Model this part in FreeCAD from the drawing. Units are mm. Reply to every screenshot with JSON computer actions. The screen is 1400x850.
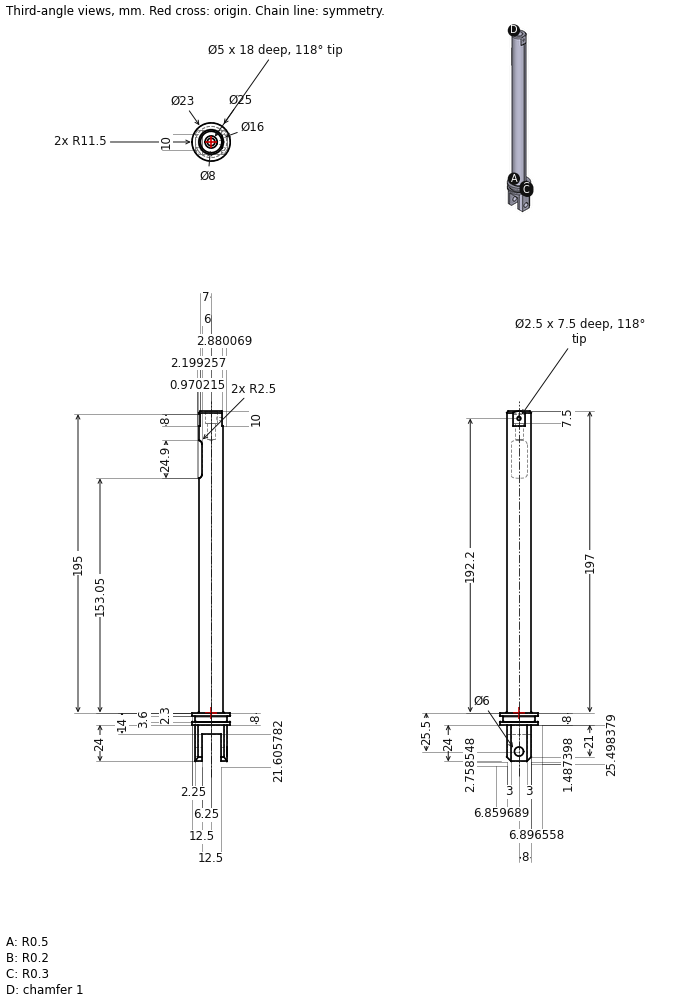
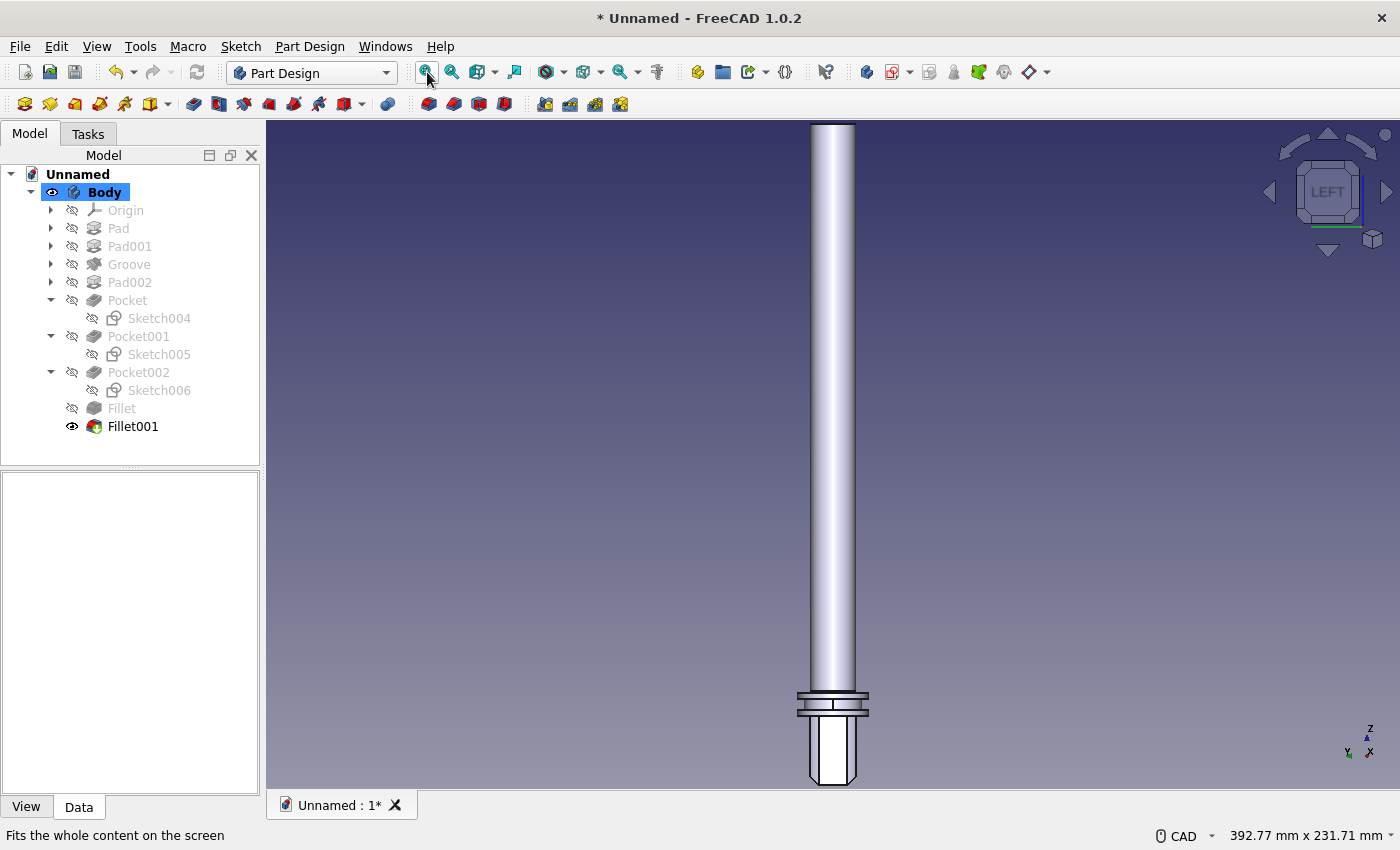
{"action": "key", "text": "v 3"}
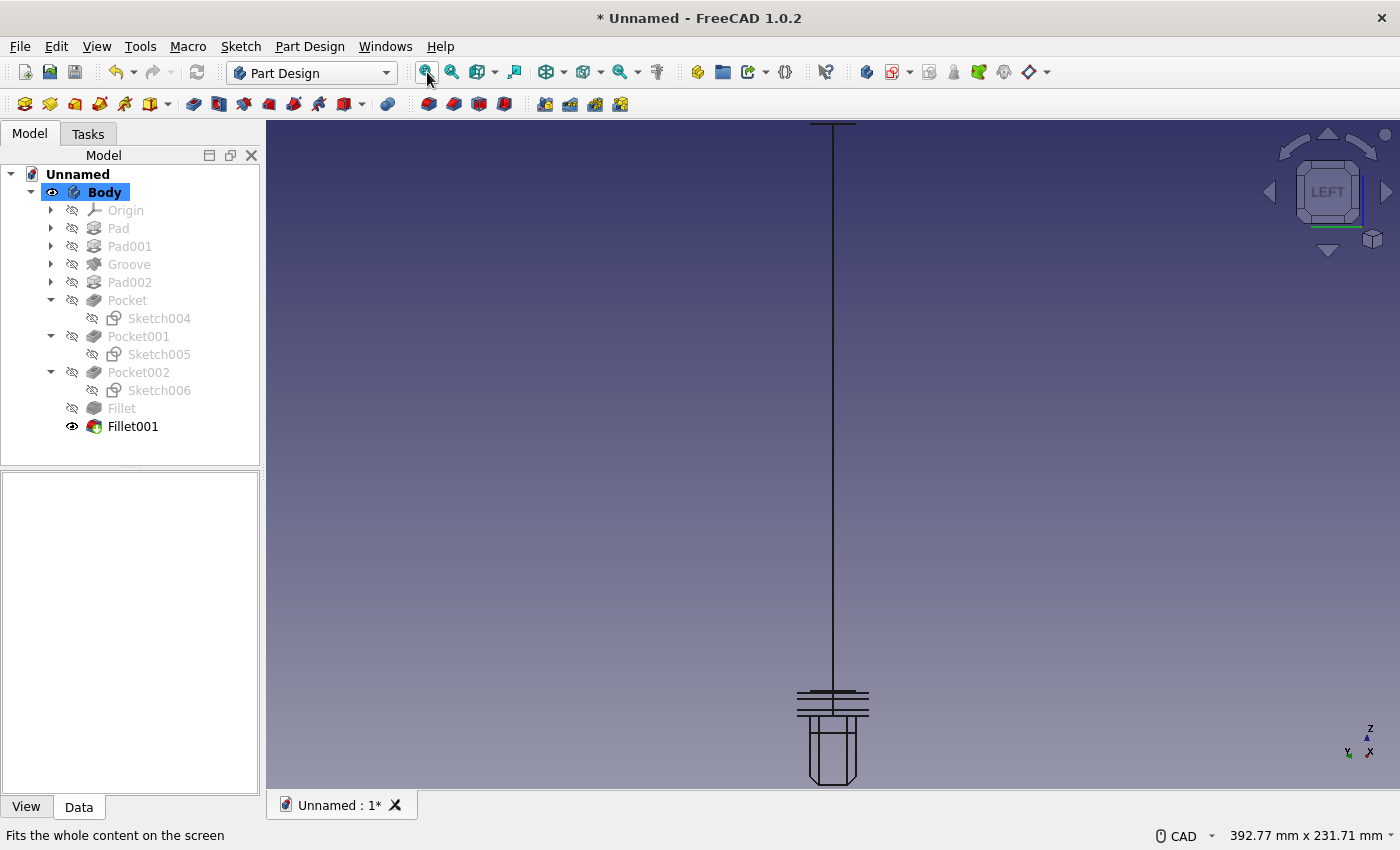
{"action": "key", "text": "0"}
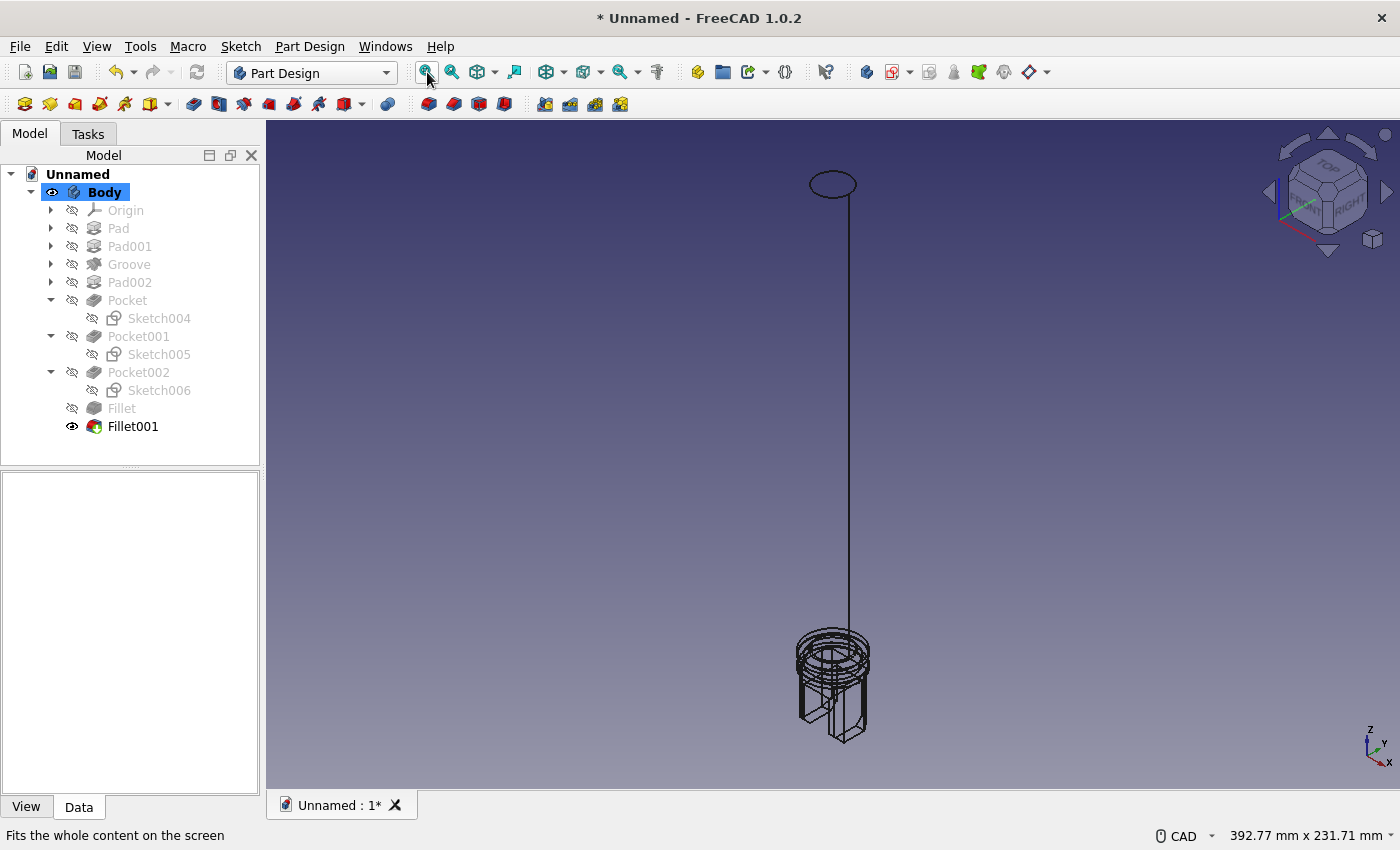
{"action": "left_click", "coordinate": [832, 645]}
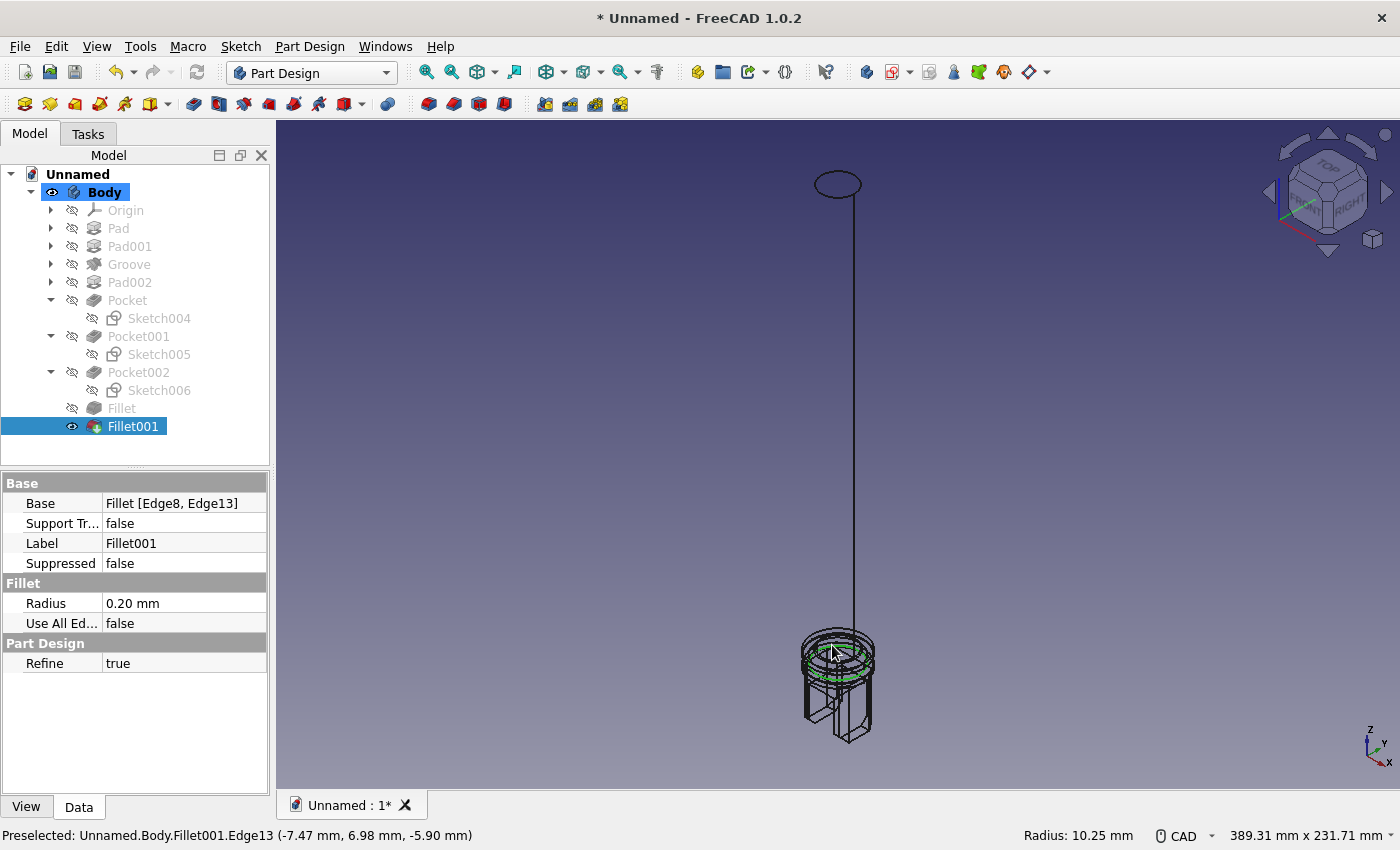
{"action": "scroll", "coordinate": [859, 665], "scroll_direction": "up", "scroll_amount": 6}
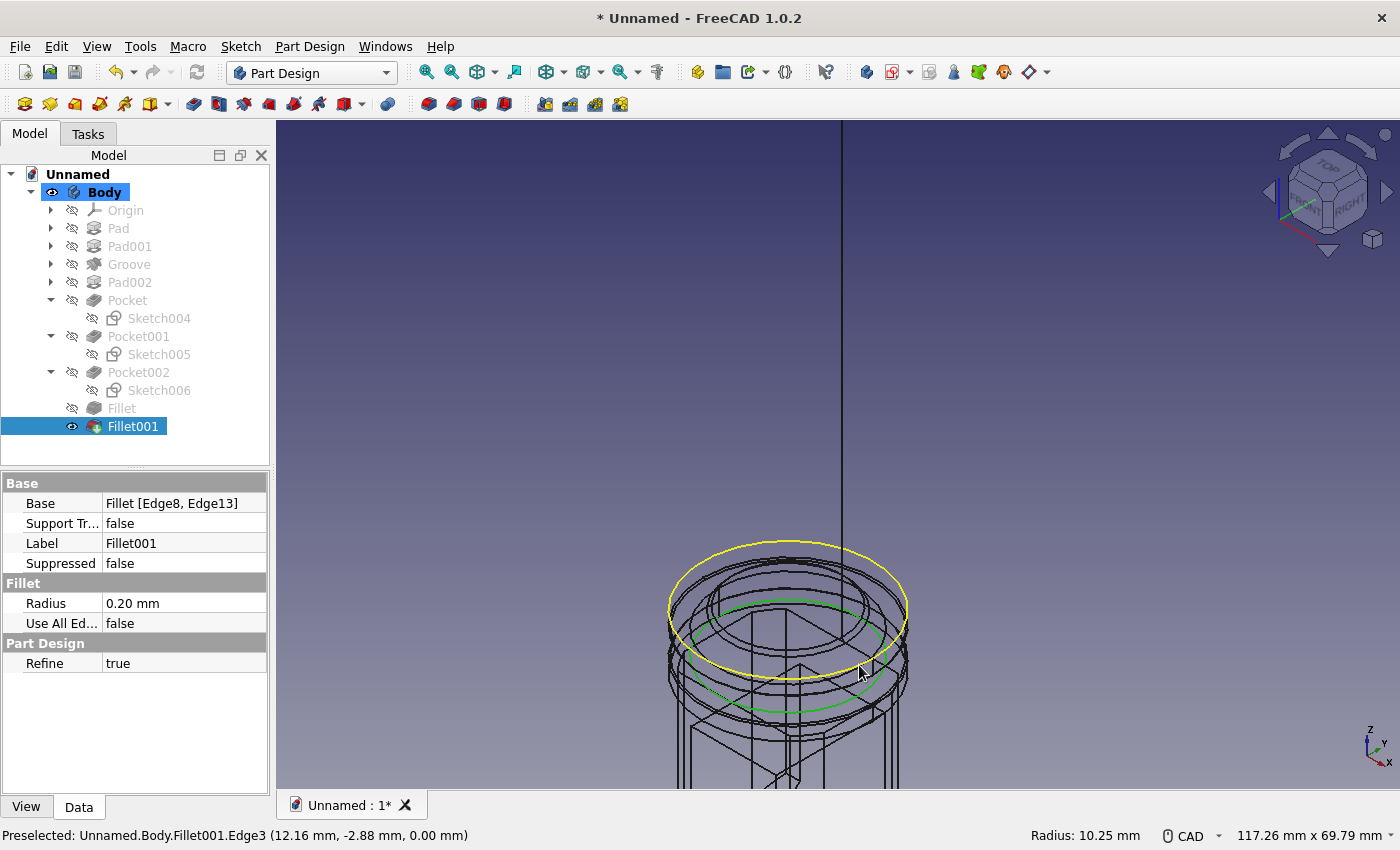
{"action": "left_click", "coordinate": [885, 636], "text": "ctrl"}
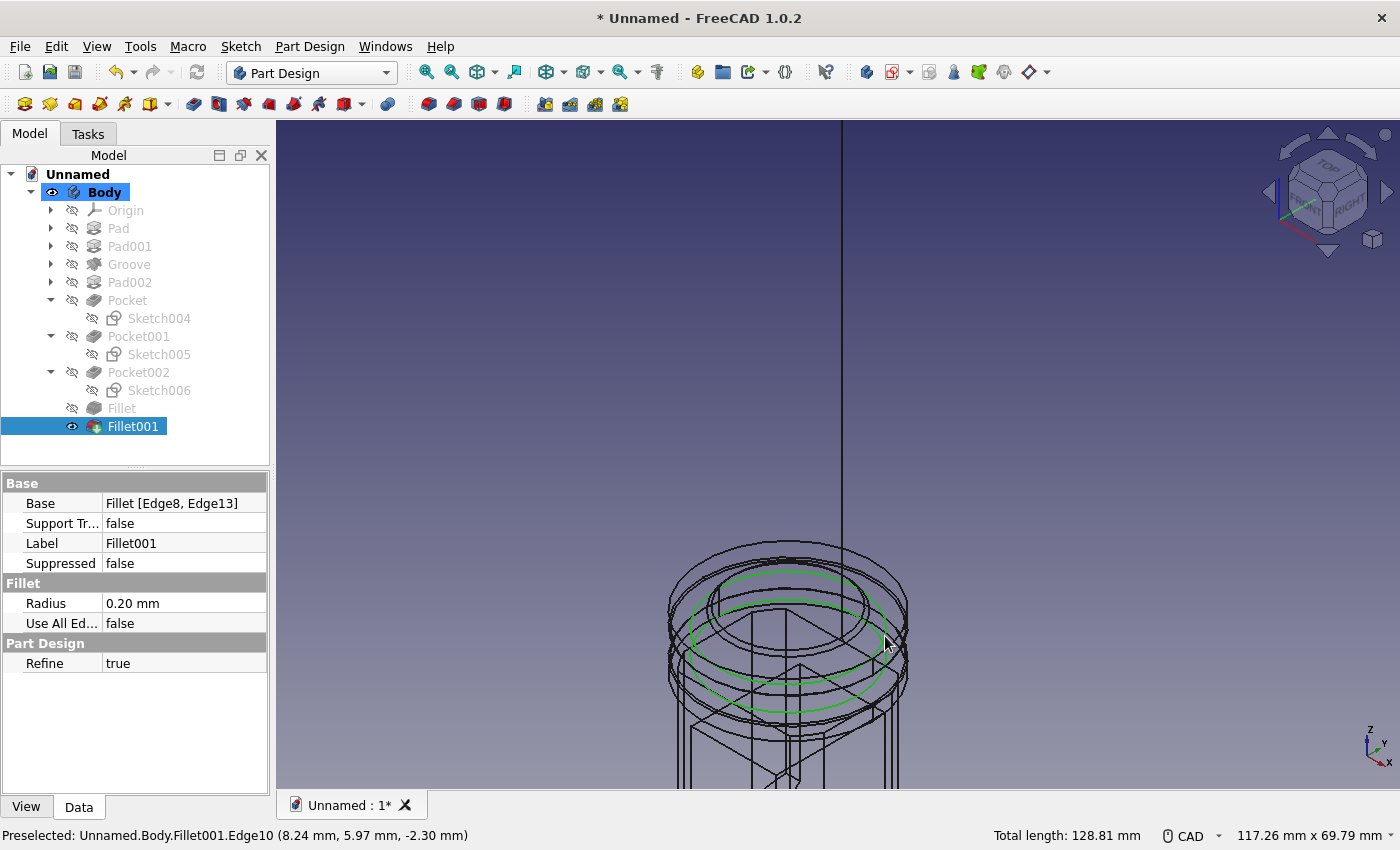
{"action": "key", "text": "v 1"}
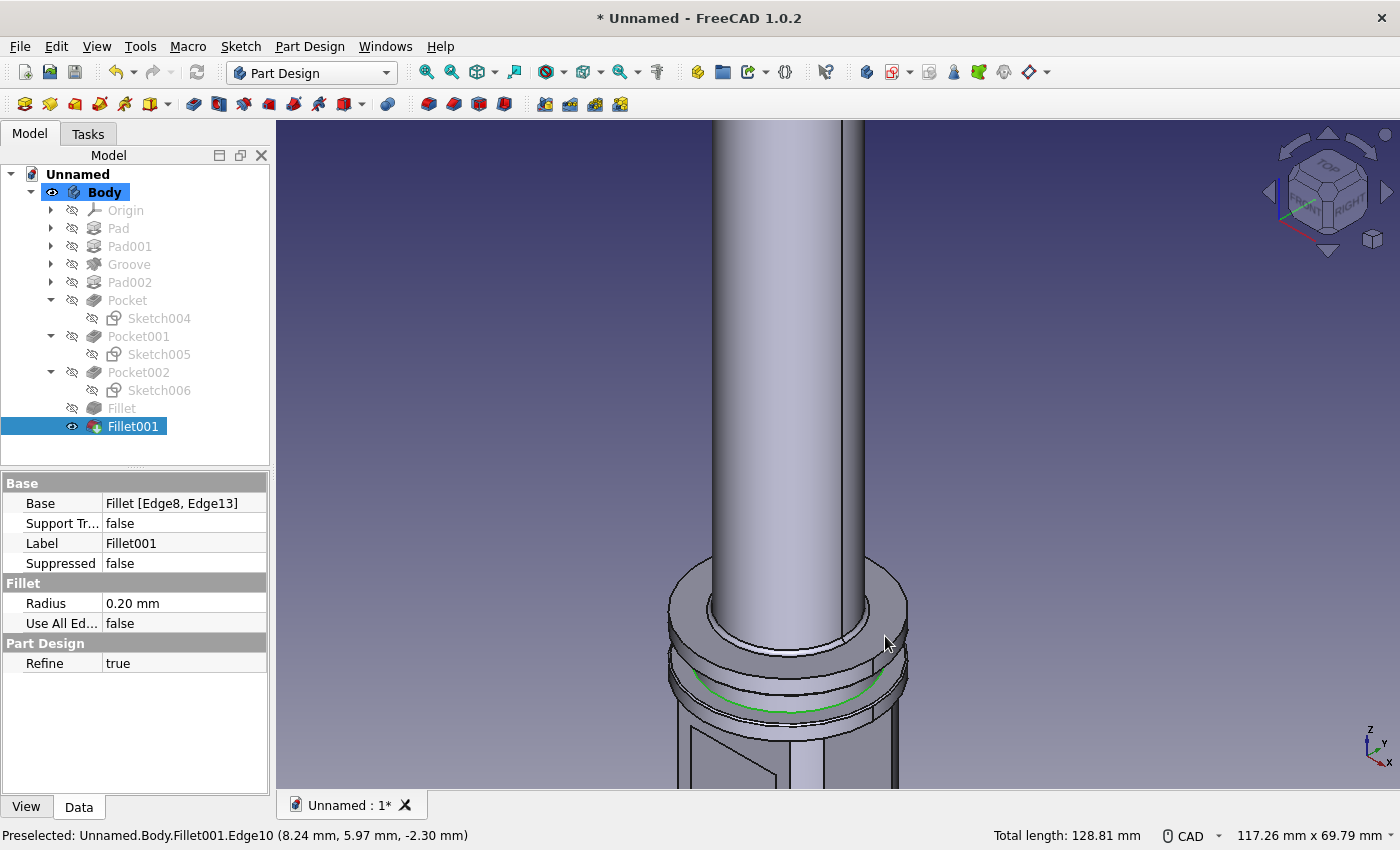
{"action": "left_click", "coordinate": [429, 104]}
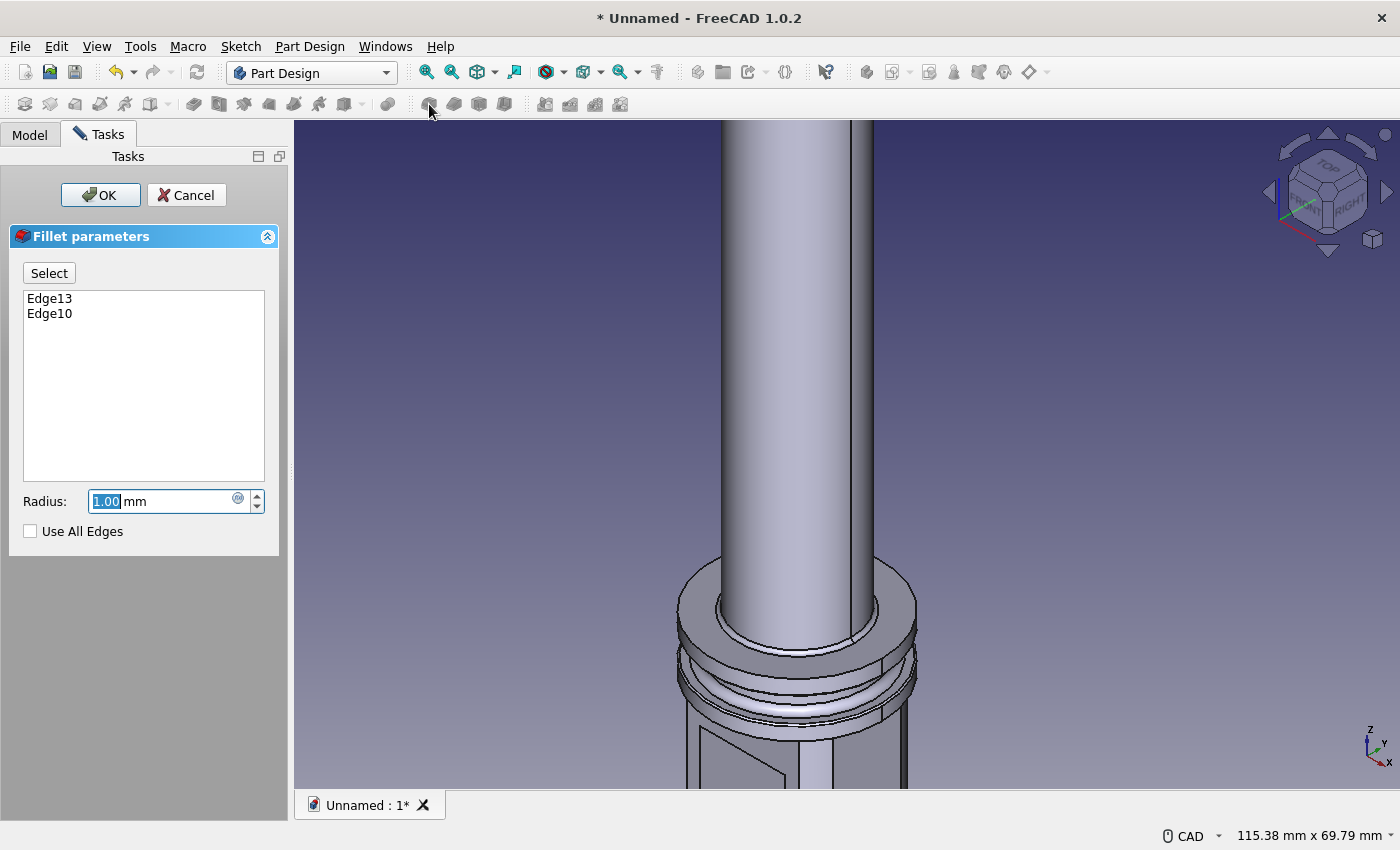
{"action": "type", "text": "0.3"}
{"action": "key", "text": "Tab"}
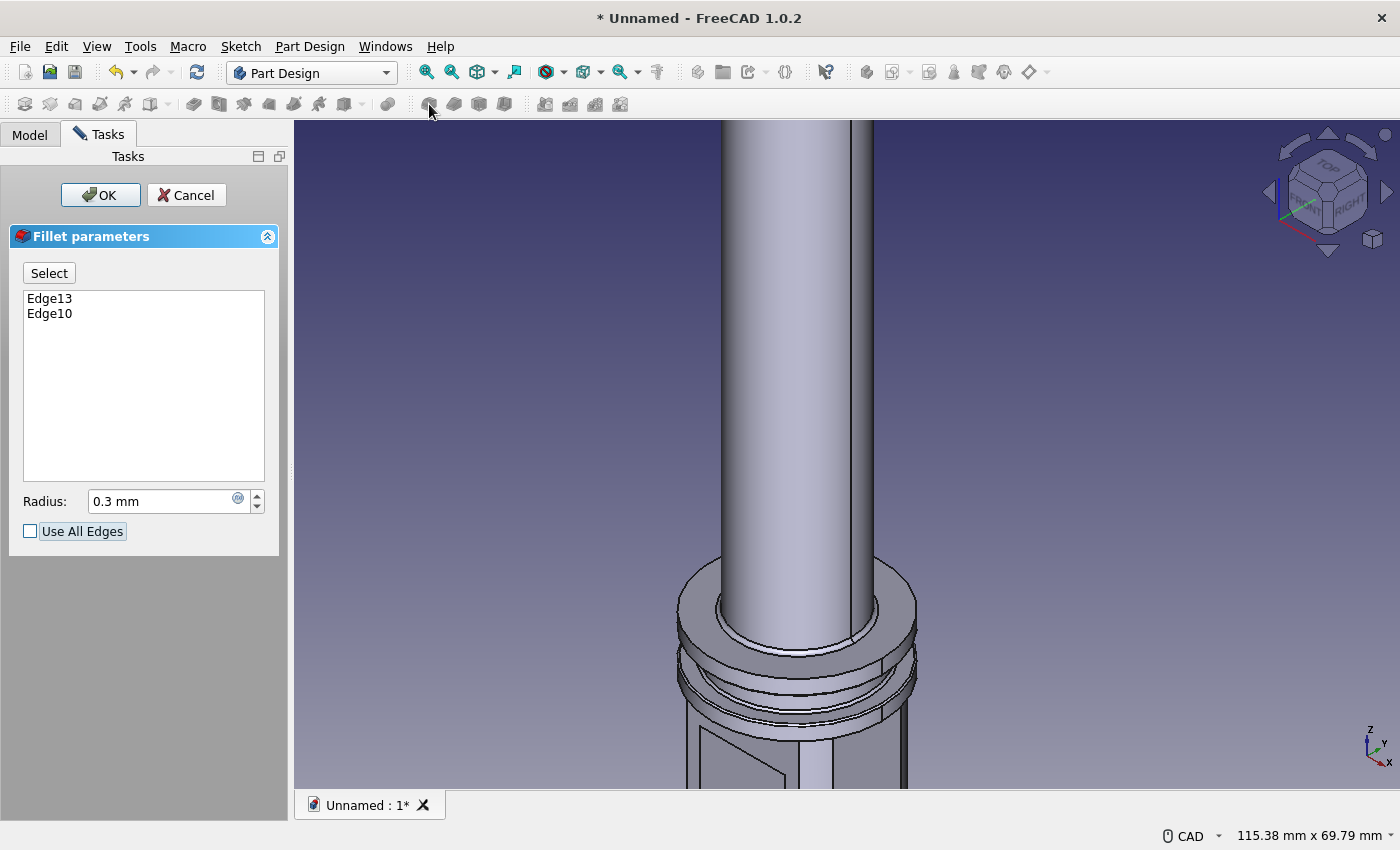
{"action": "left_click", "coordinate": [101, 195]}